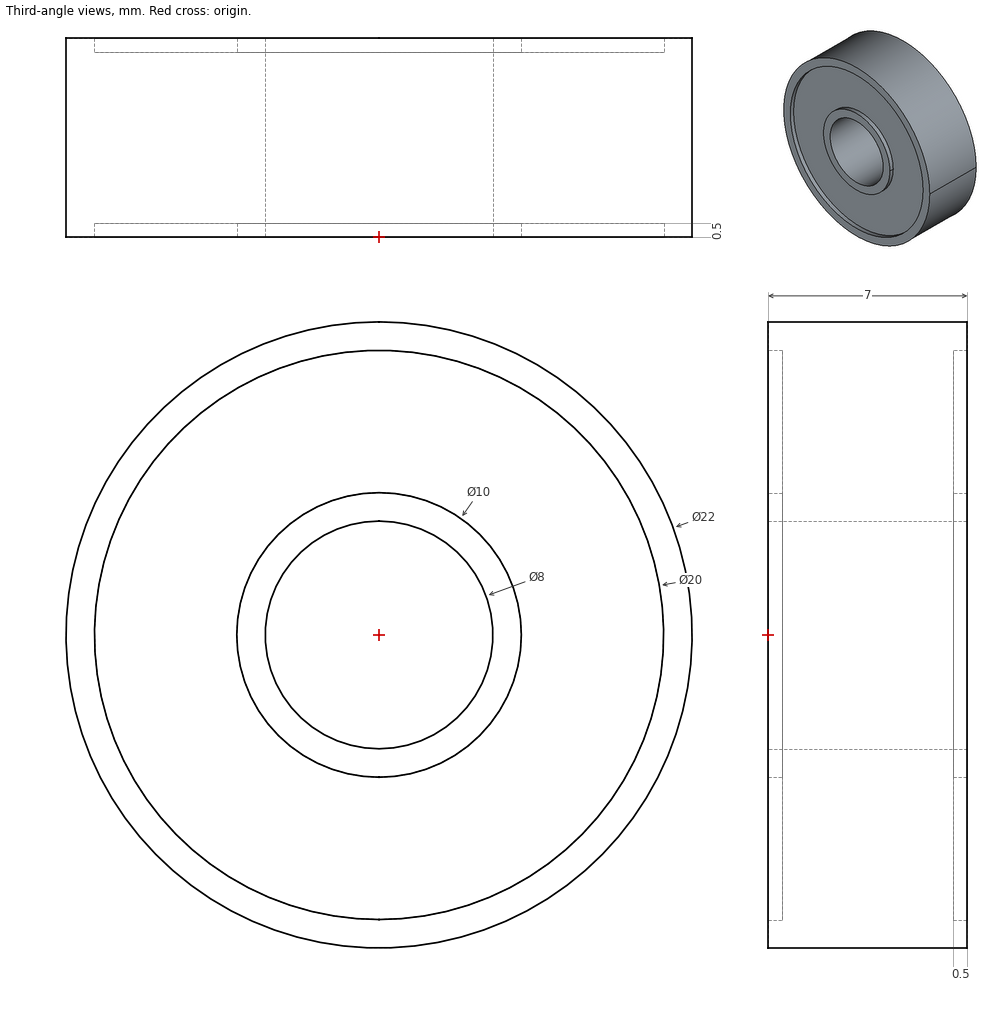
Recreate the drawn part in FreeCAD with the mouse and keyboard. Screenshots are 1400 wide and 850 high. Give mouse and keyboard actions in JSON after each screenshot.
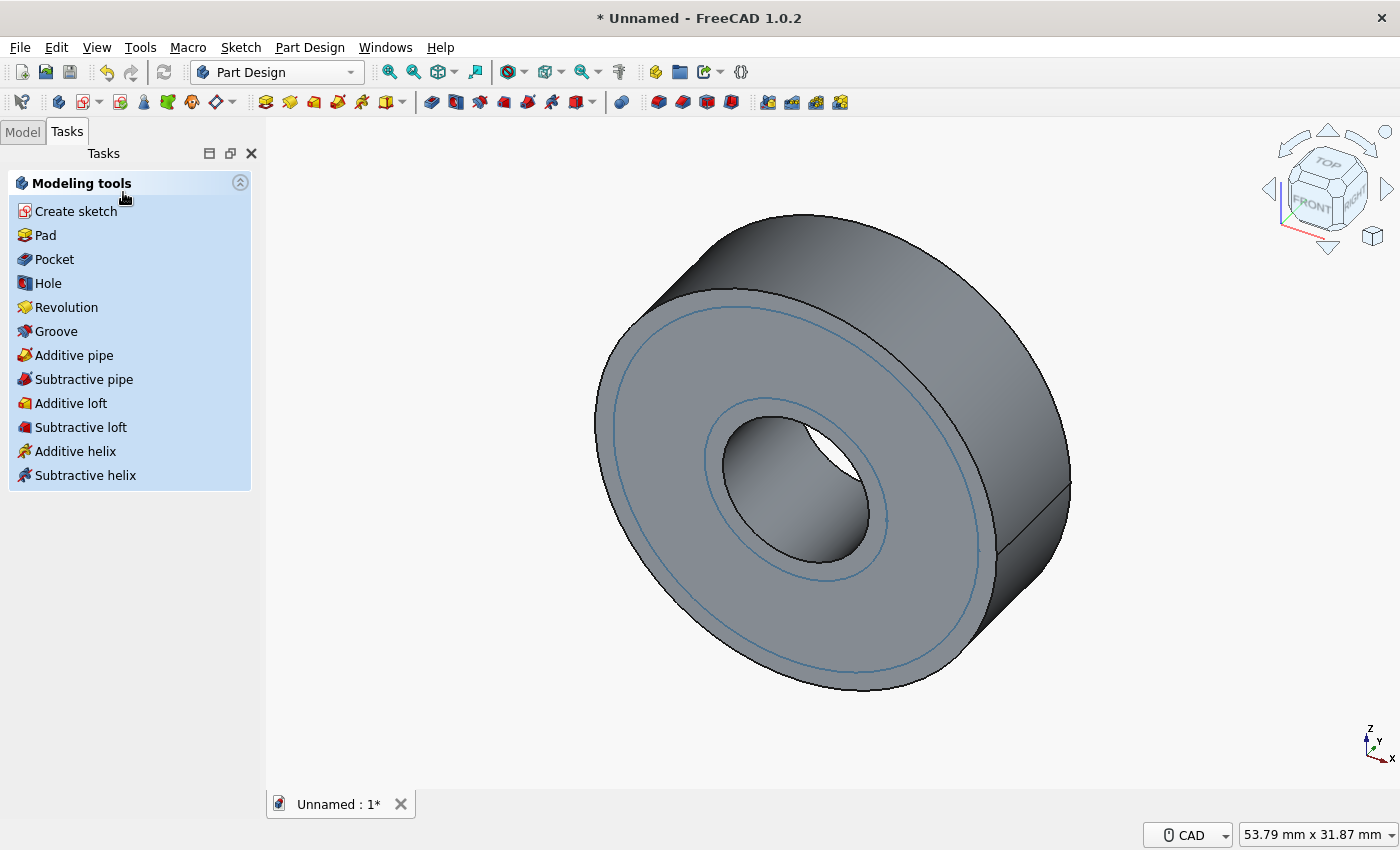
{"action": "left_click", "coordinate": [432, 102]}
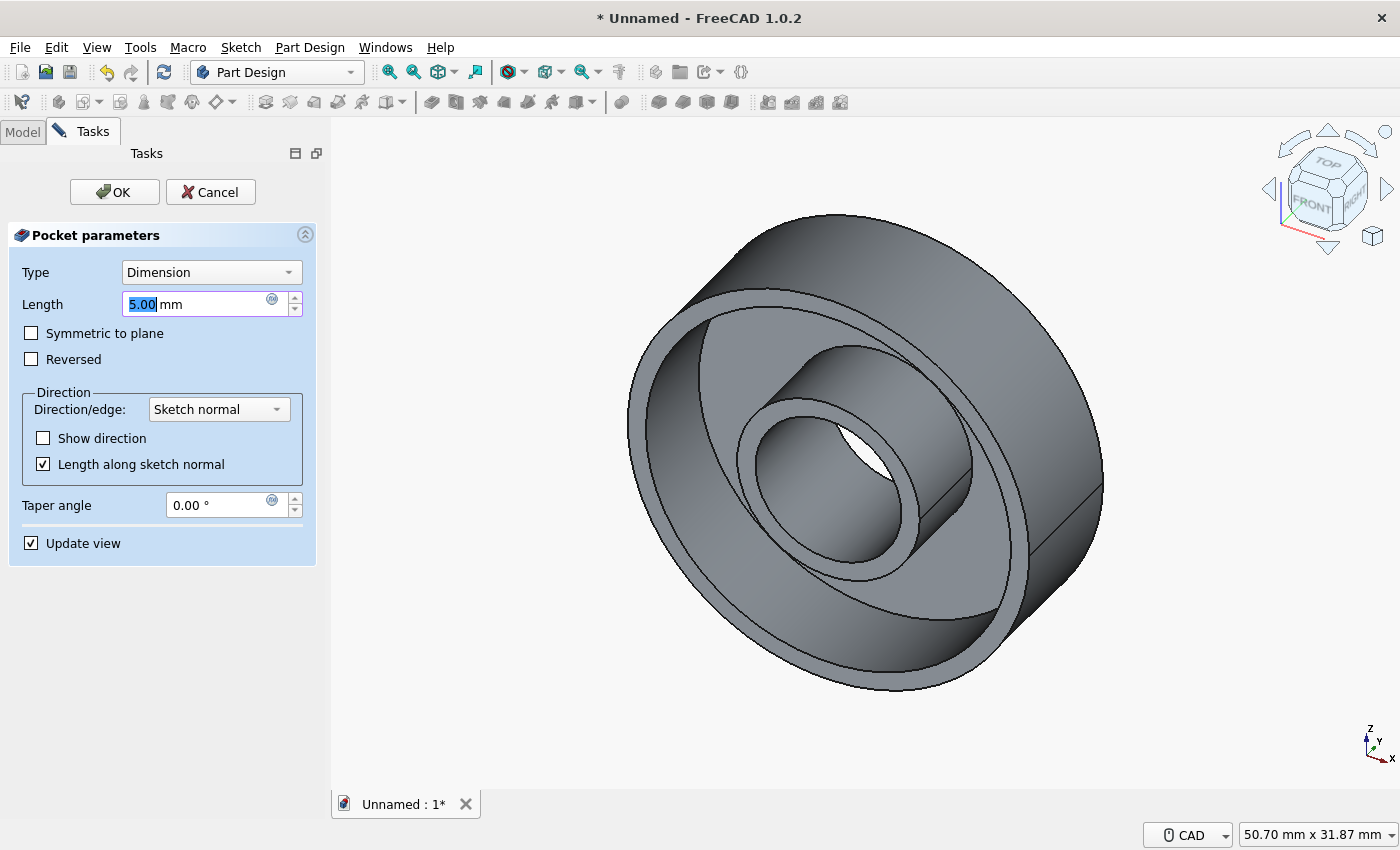
{"action": "type", "text": "0.5"}
{"action": "key", "text": "Tab"}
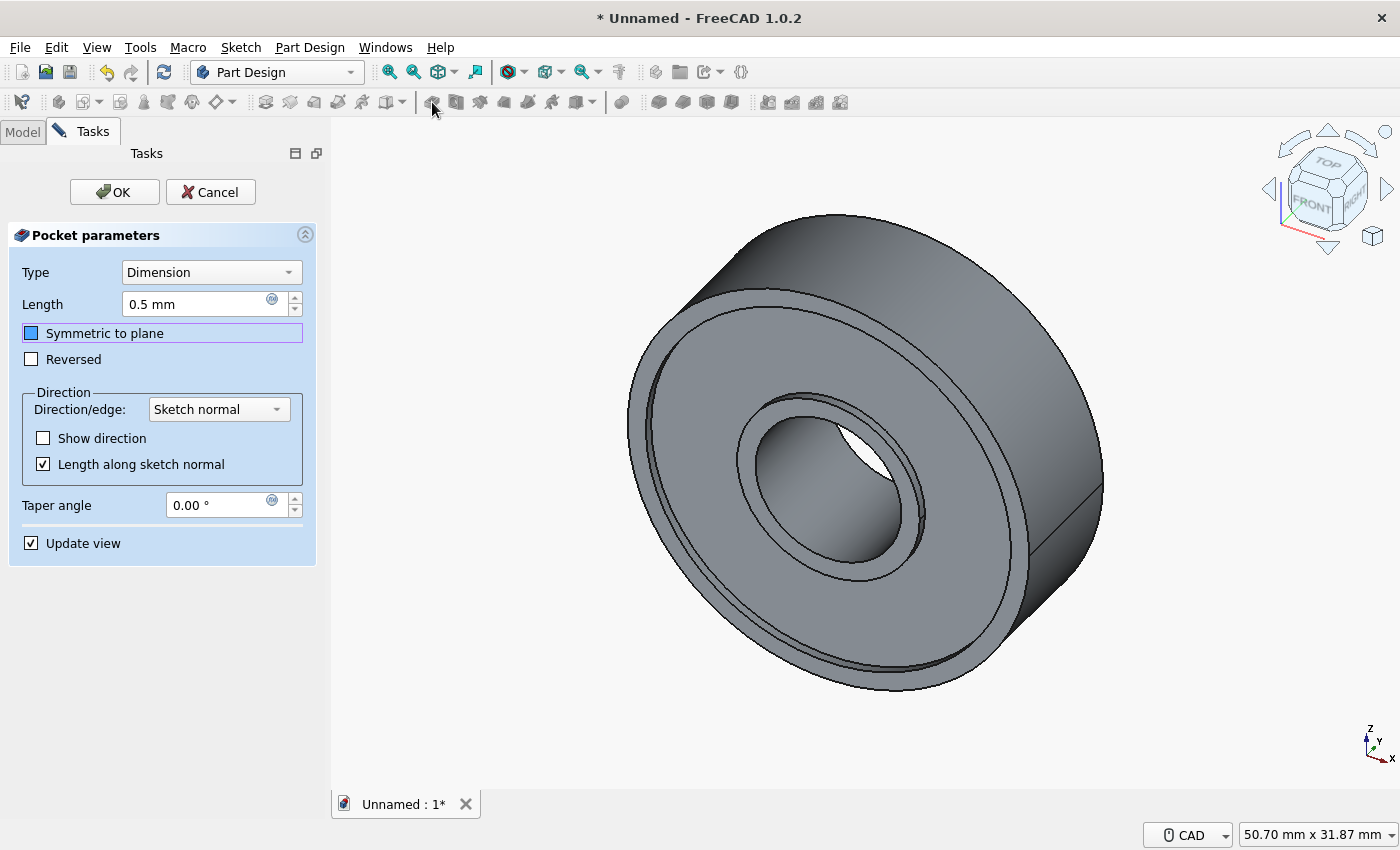
{"action": "left_click", "coordinate": [115, 192]}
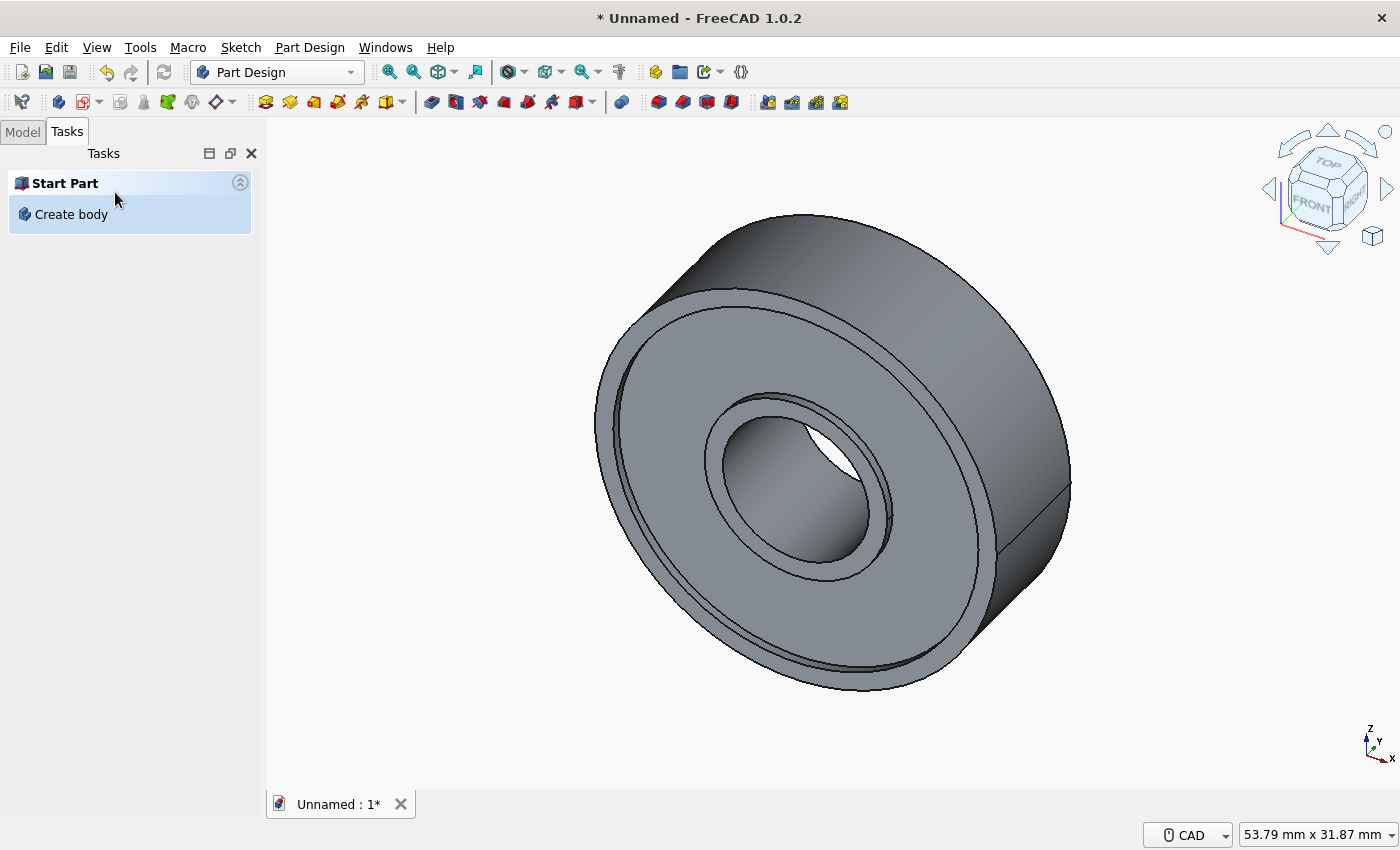
{"action": "left_click", "coordinate": [23, 131]}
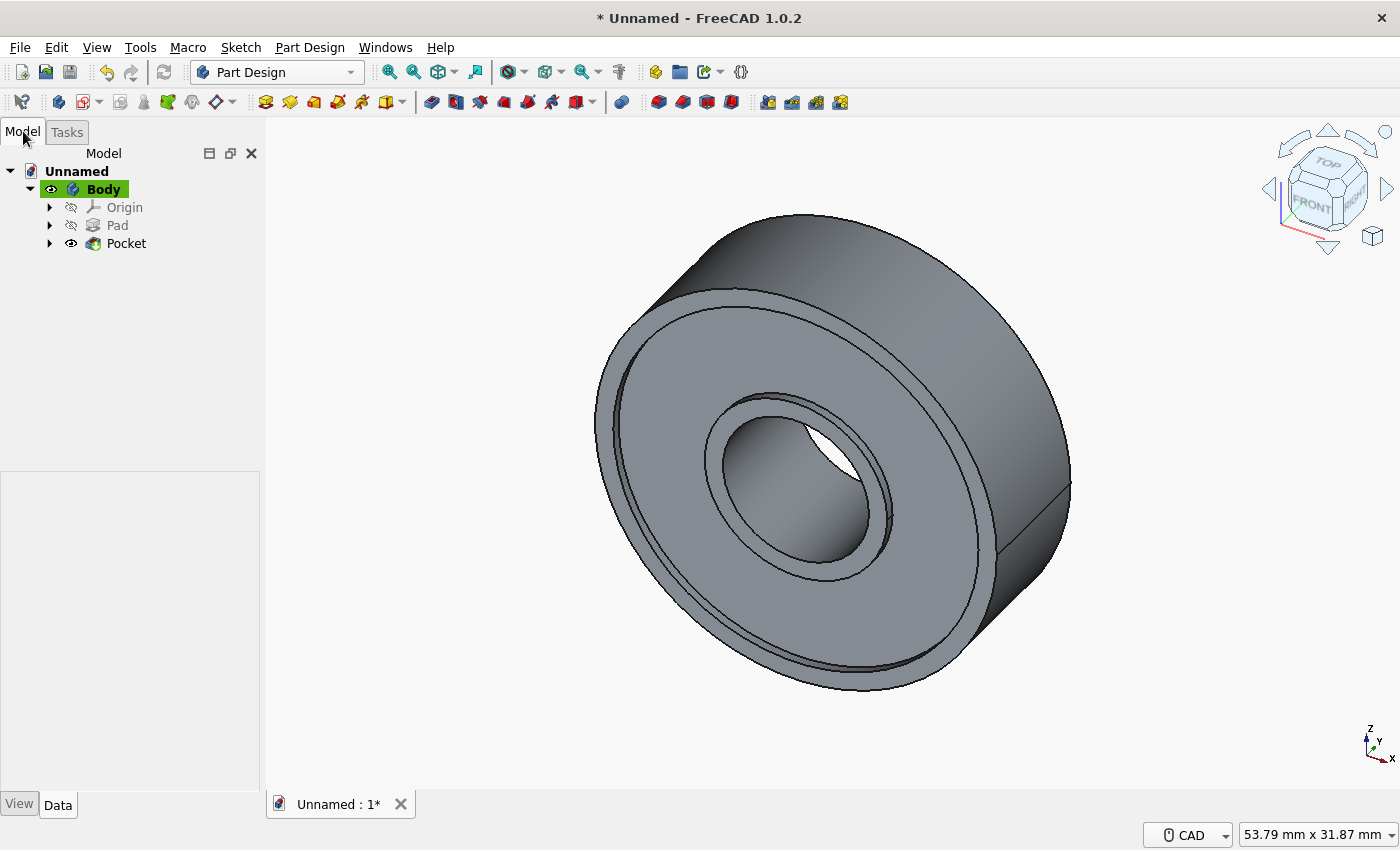
{"action": "left_click", "coordinate": [50, 207]}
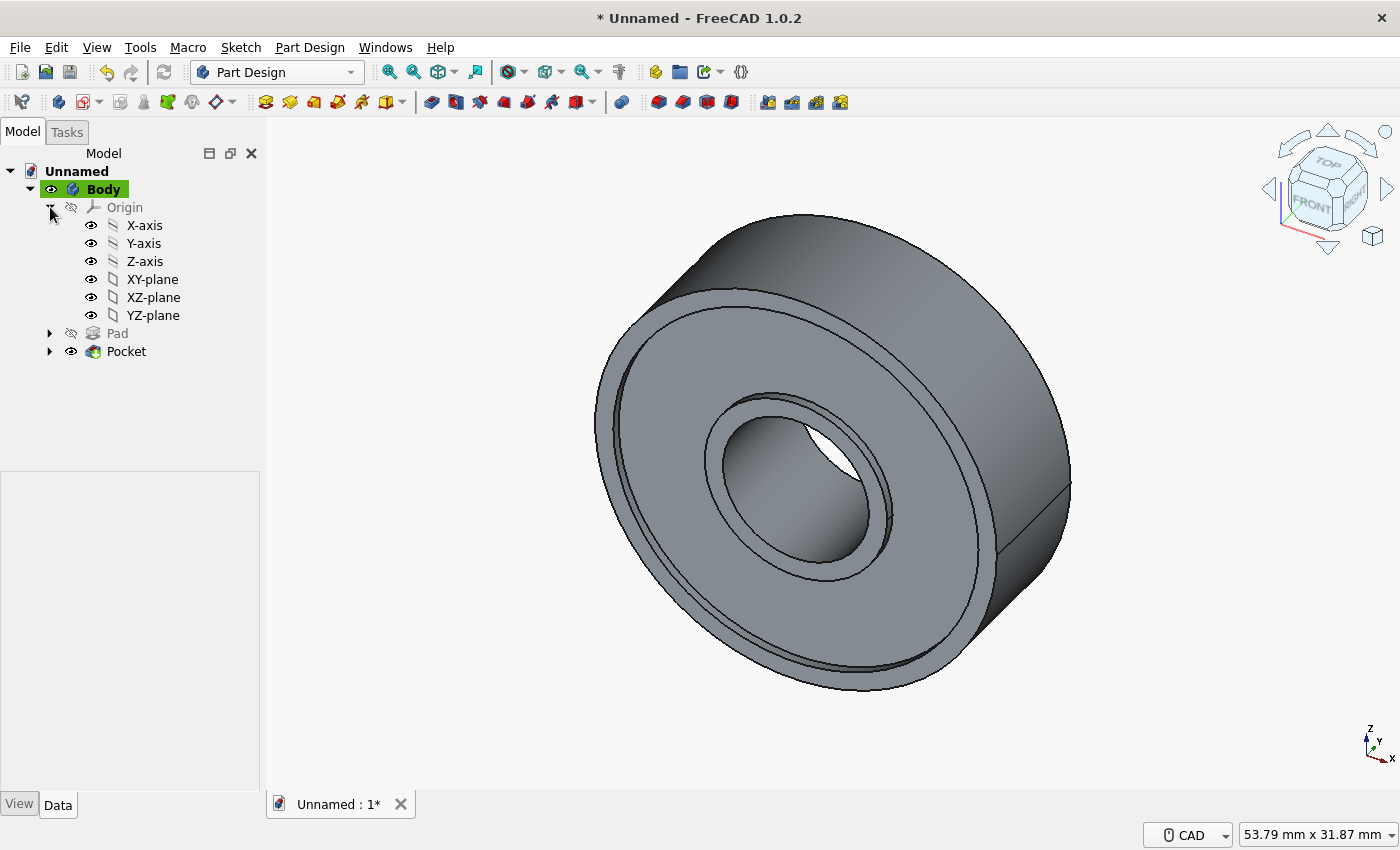
{"action": "left_click", "coordinate": [136, 297]}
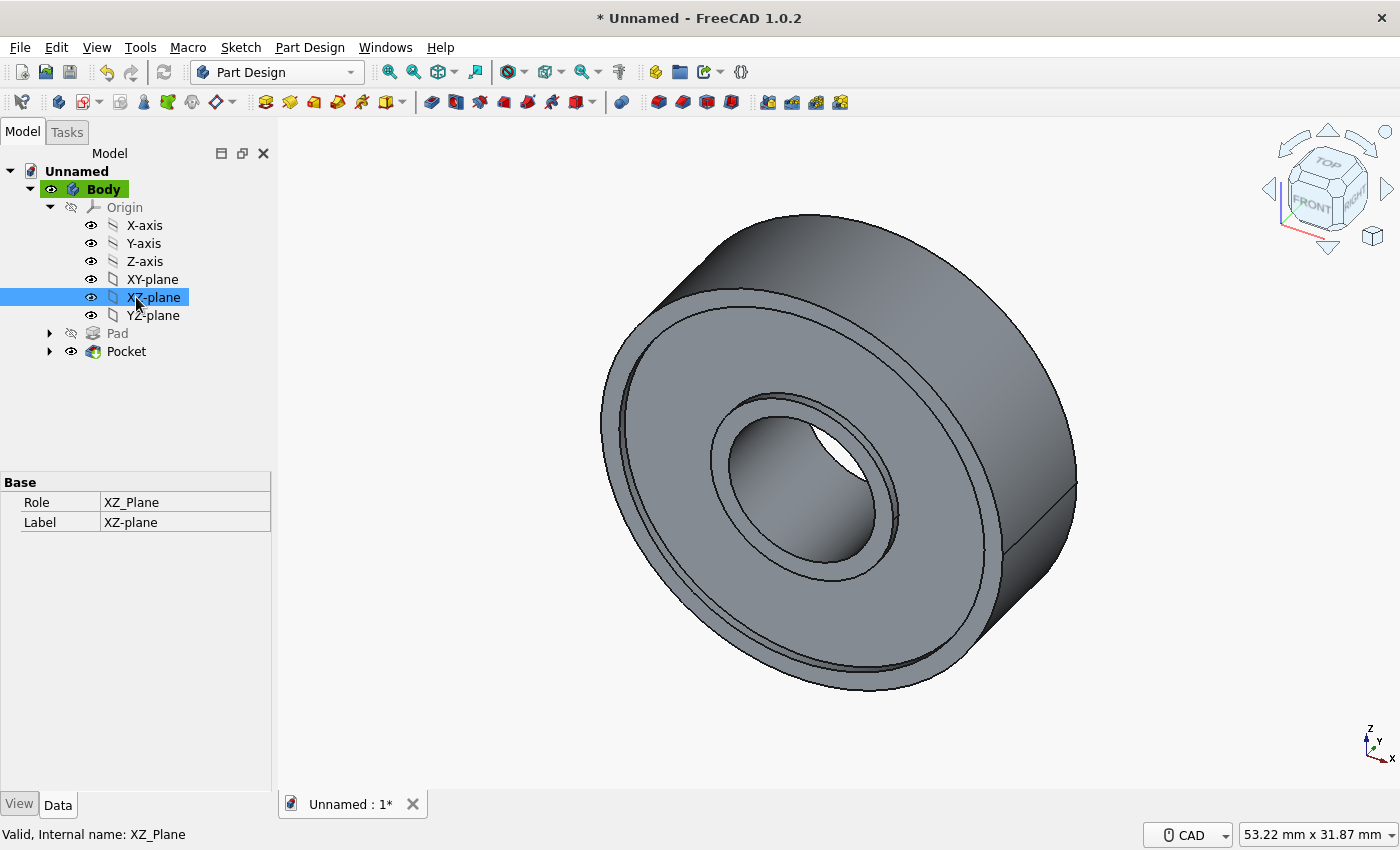
{"action": "left_click", "coordinate": [216, 102]}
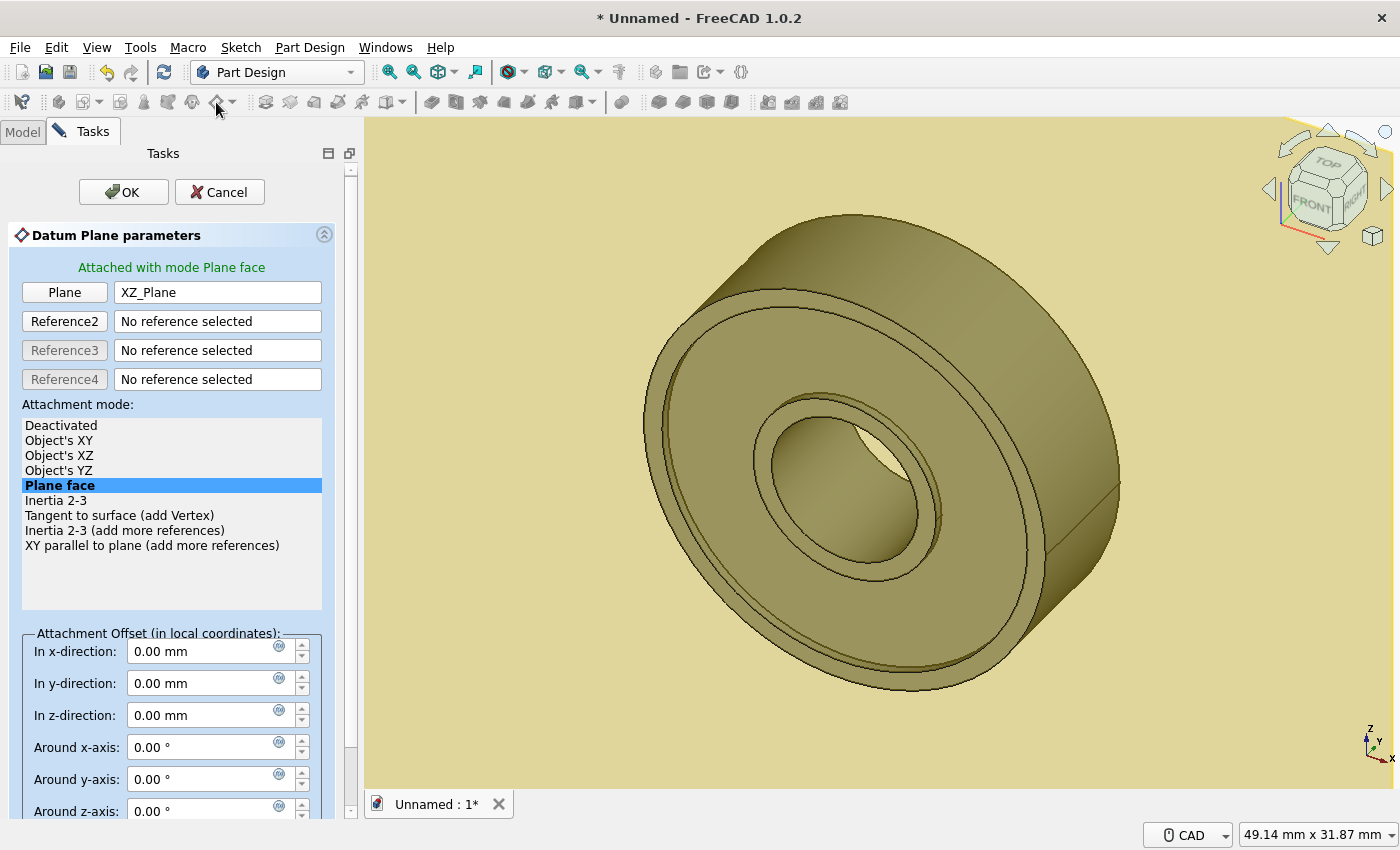
{"action": "triple_click", "coordinate": [210, 715]}